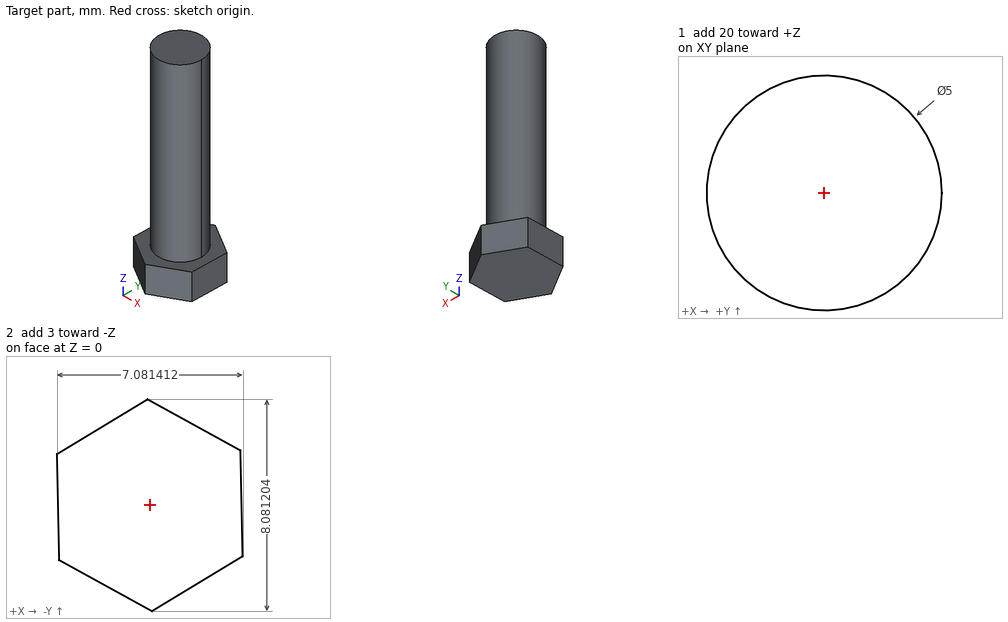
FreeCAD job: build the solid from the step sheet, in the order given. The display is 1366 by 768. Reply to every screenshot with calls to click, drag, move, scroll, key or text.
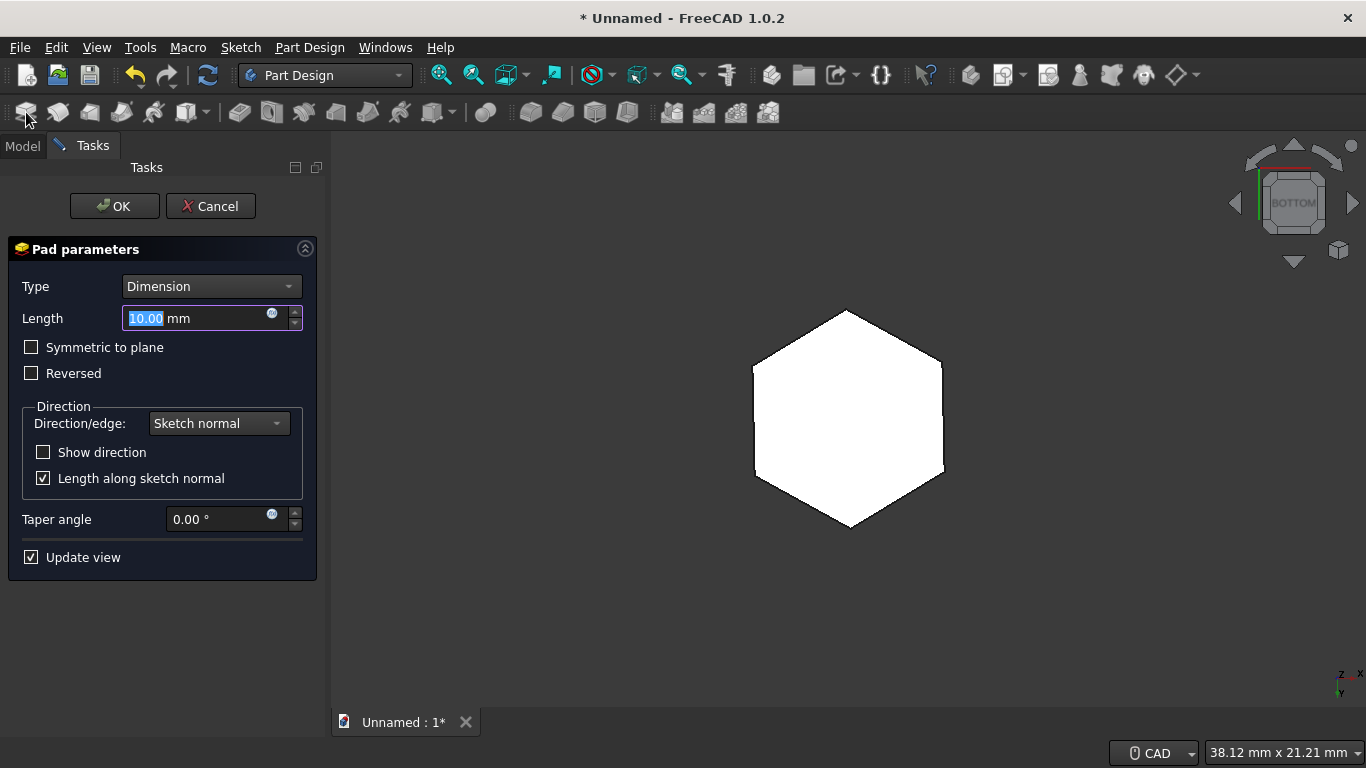
text(3)
key(Tab)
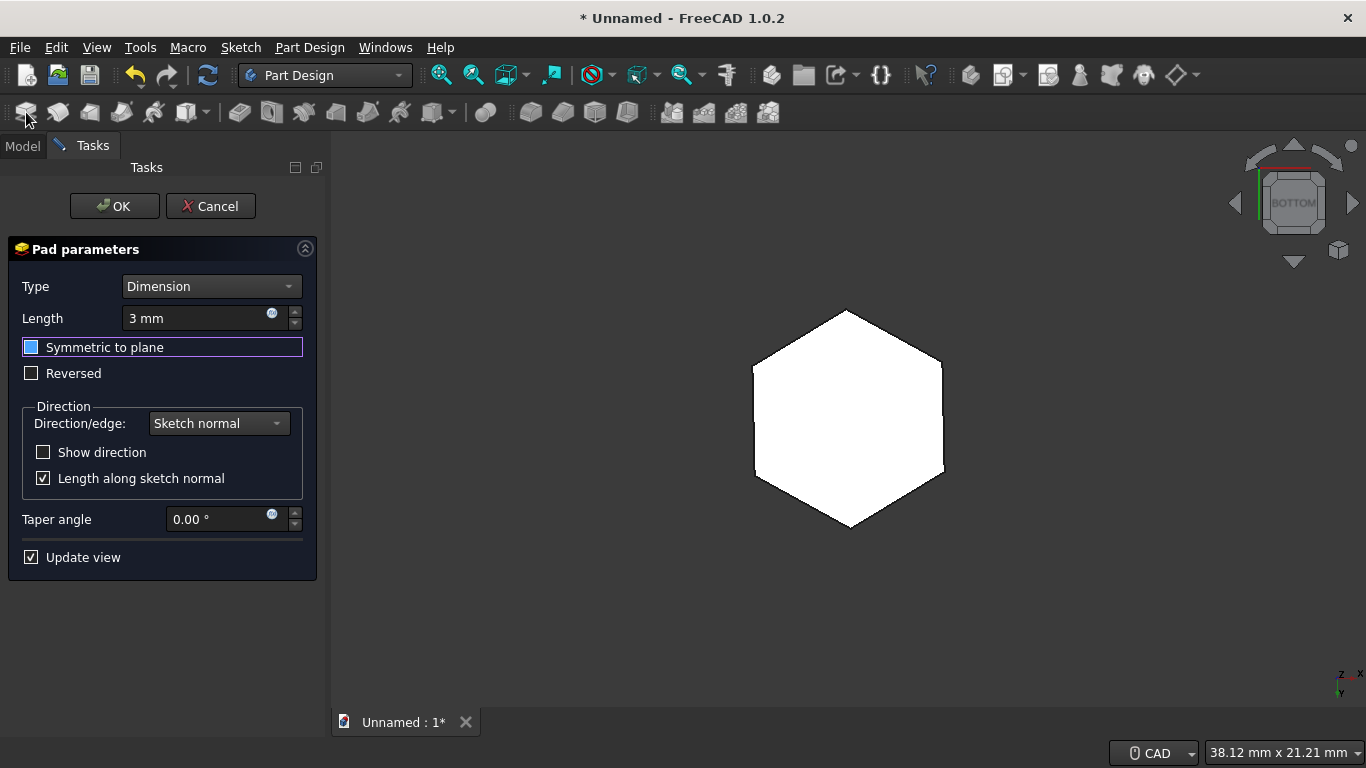
click(115, 206)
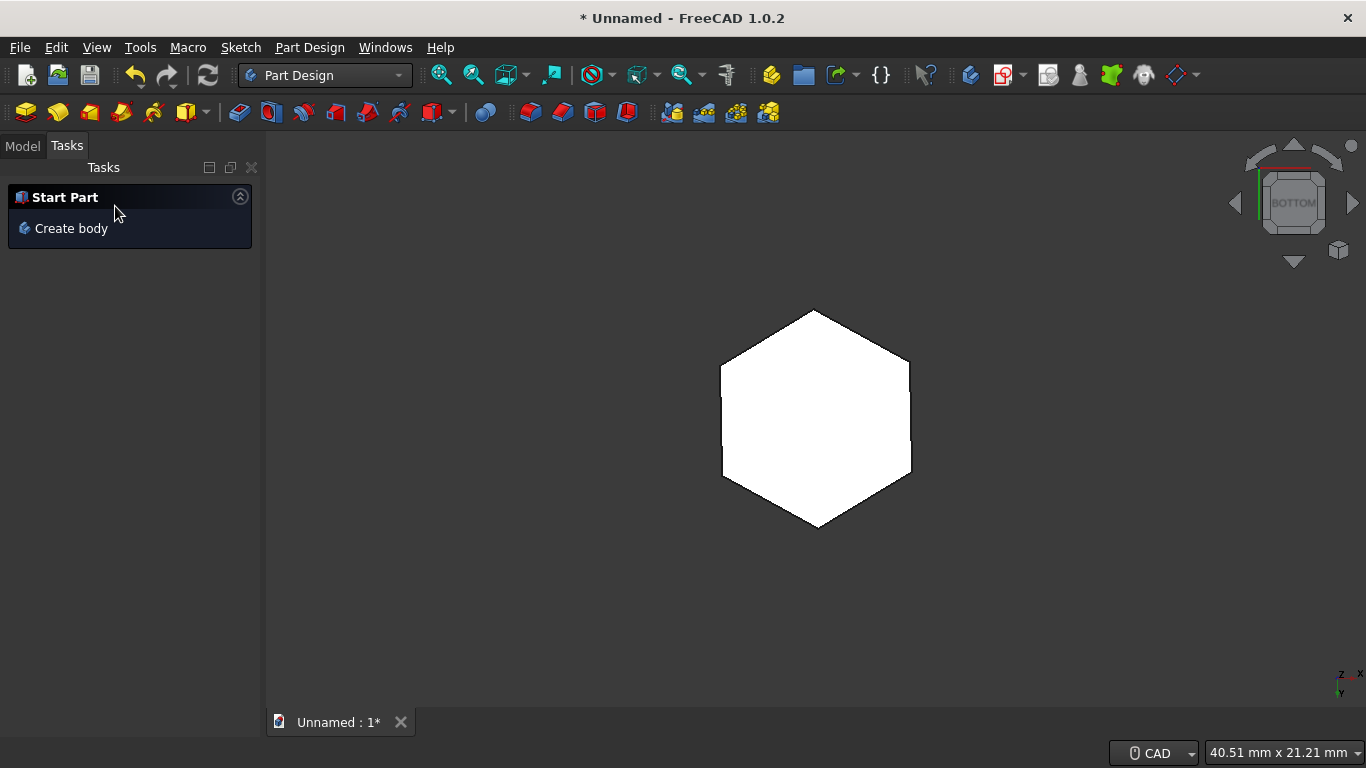
key(0)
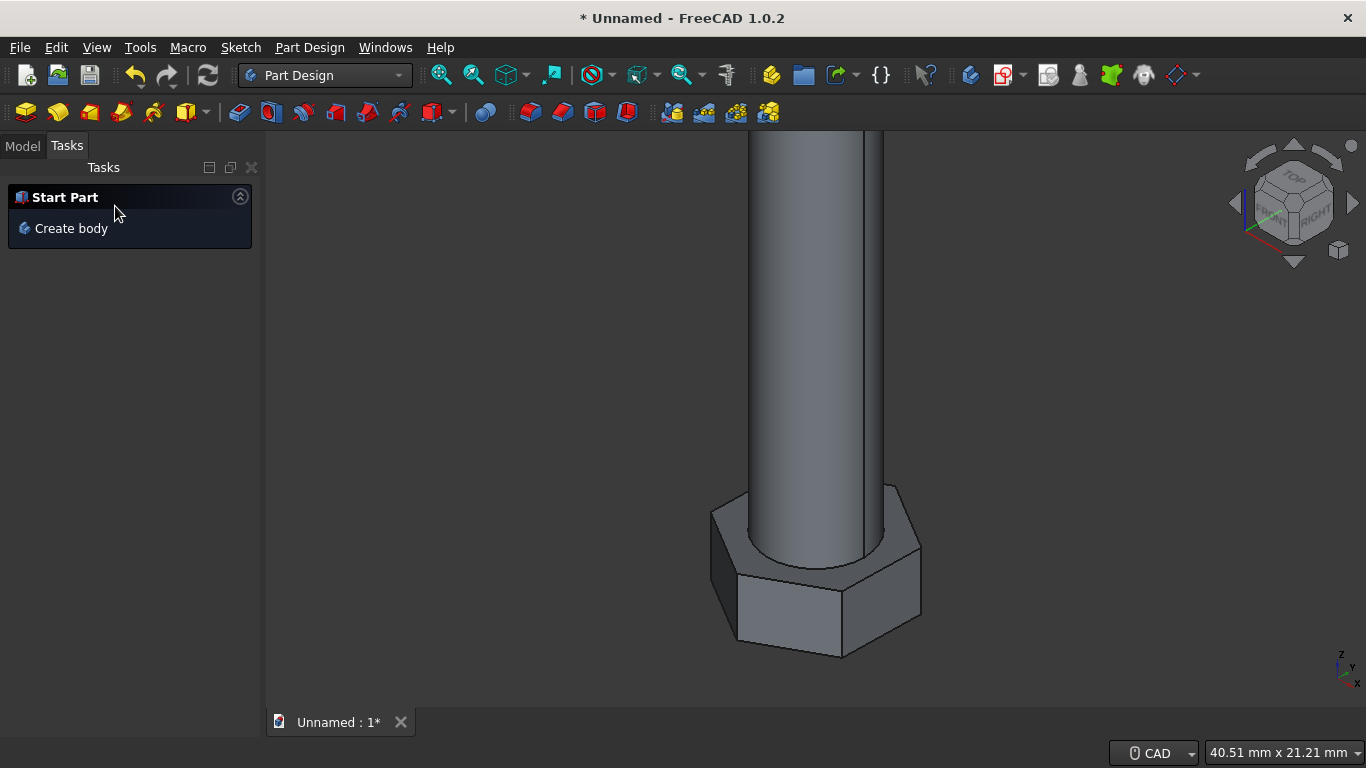
key(v)
key(f)